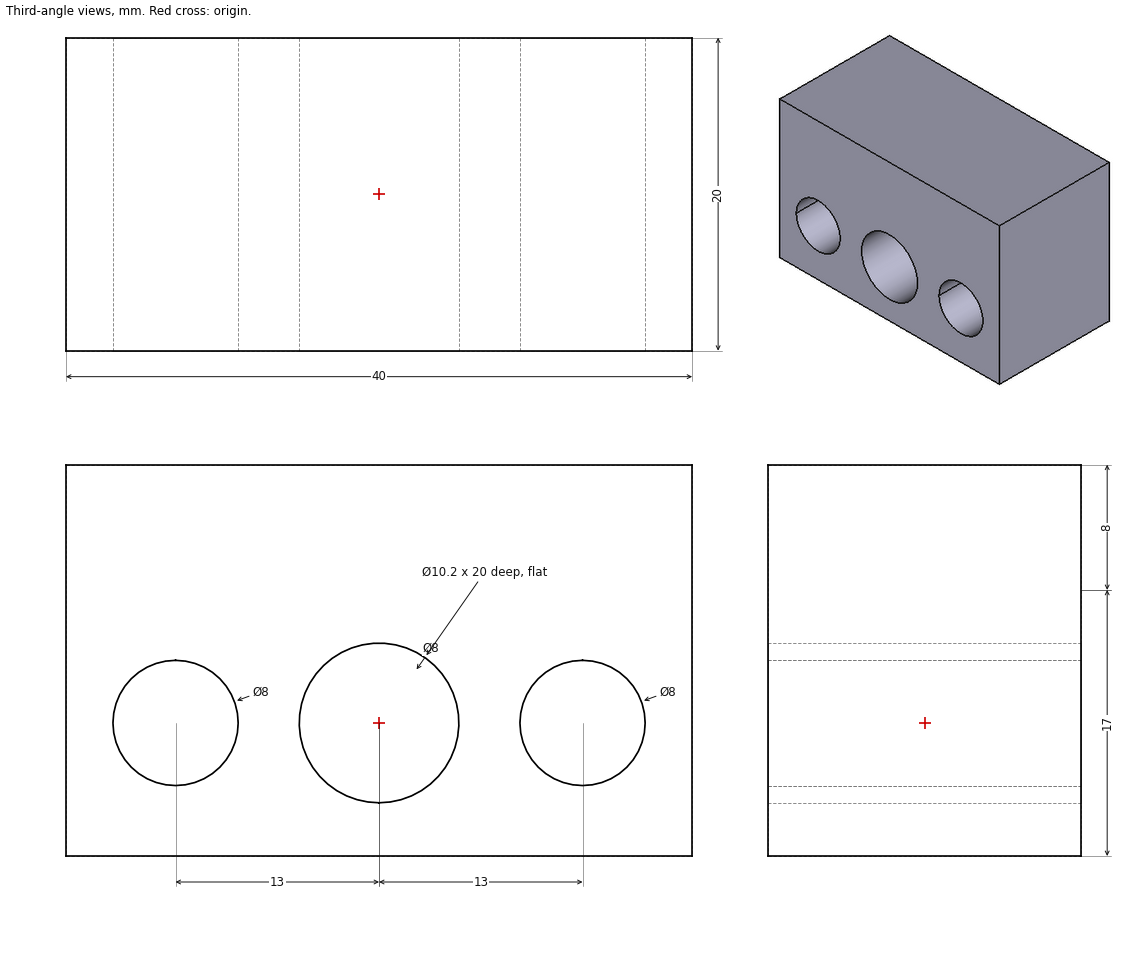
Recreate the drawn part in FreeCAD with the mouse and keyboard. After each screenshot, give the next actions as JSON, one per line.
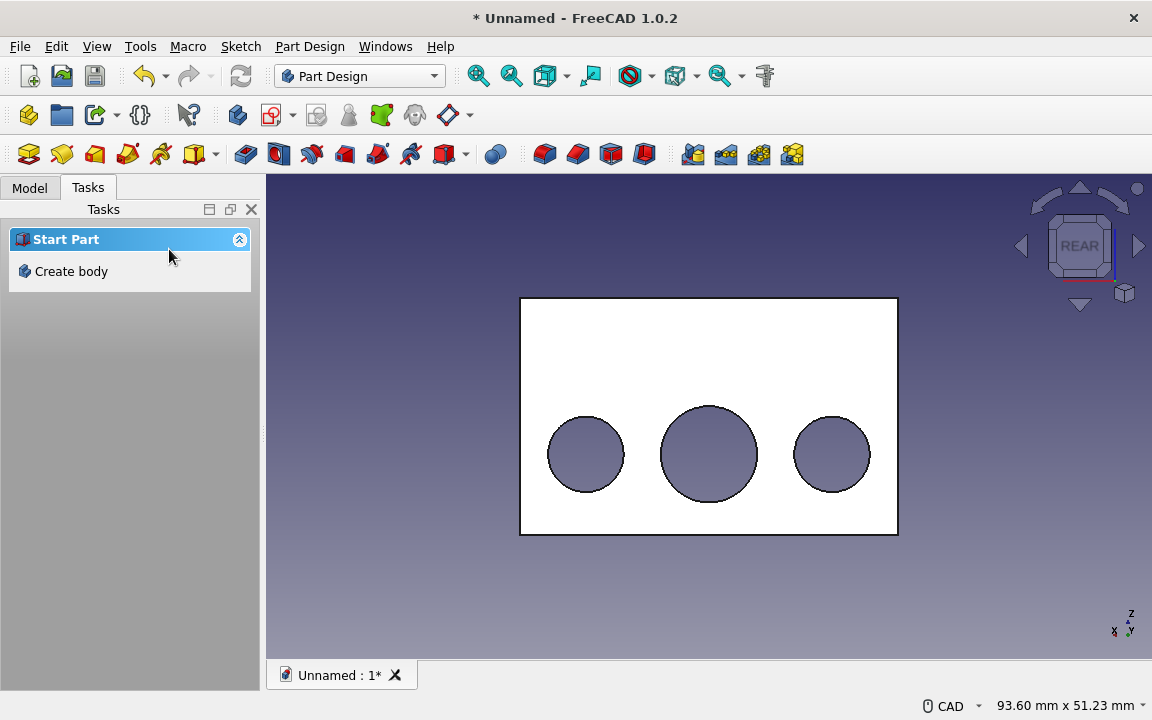
{"action": "key", "text": "0"}